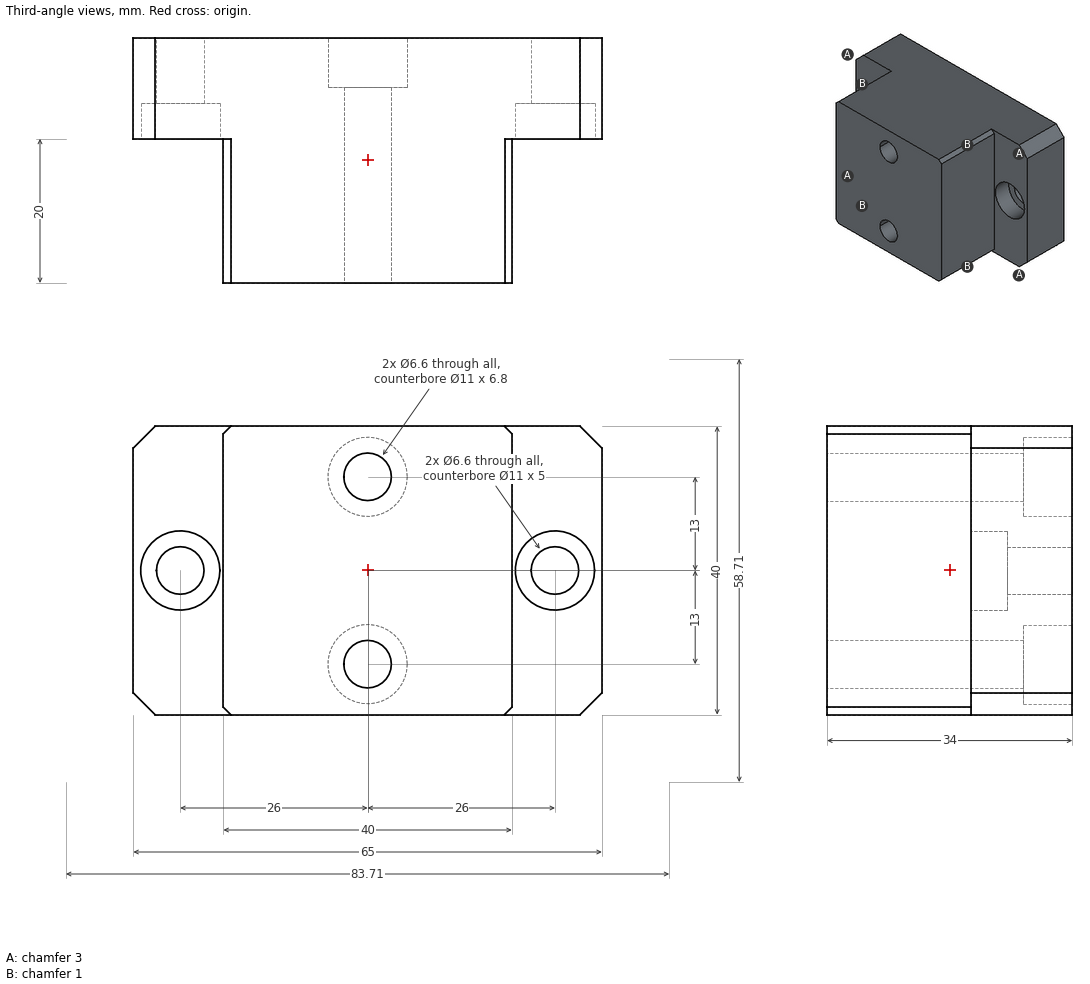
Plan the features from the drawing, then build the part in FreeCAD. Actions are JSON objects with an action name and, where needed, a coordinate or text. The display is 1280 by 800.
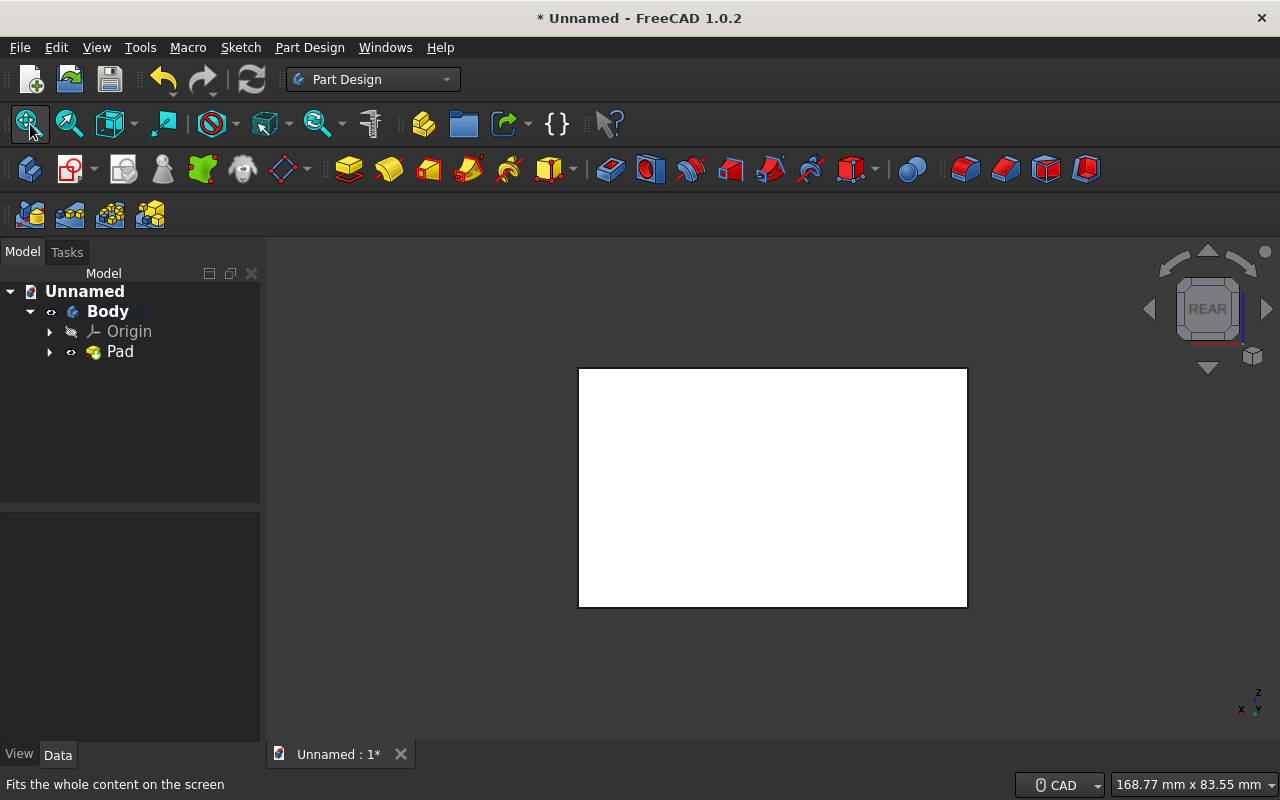
{"action": "left_click", "coordinate": [717, 487]}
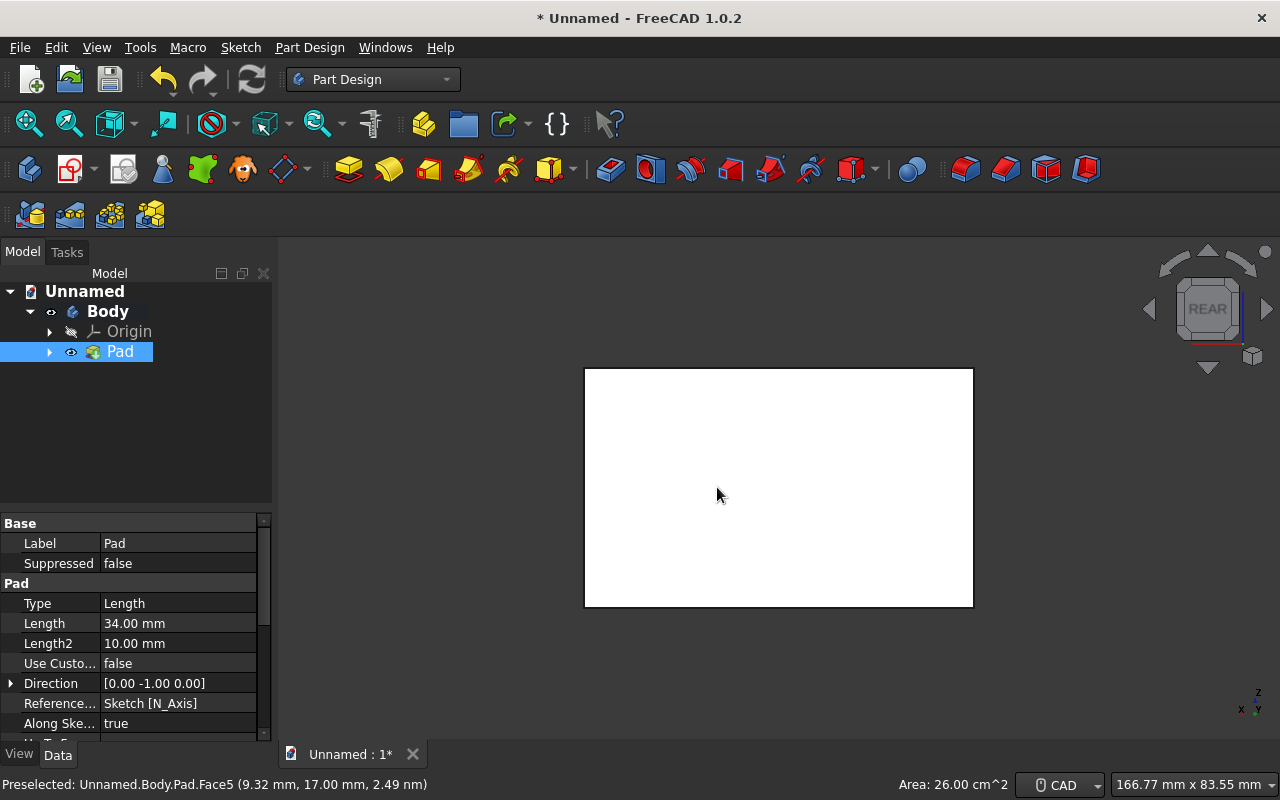
{"action": "left_click", "coordinate": [70, 170]}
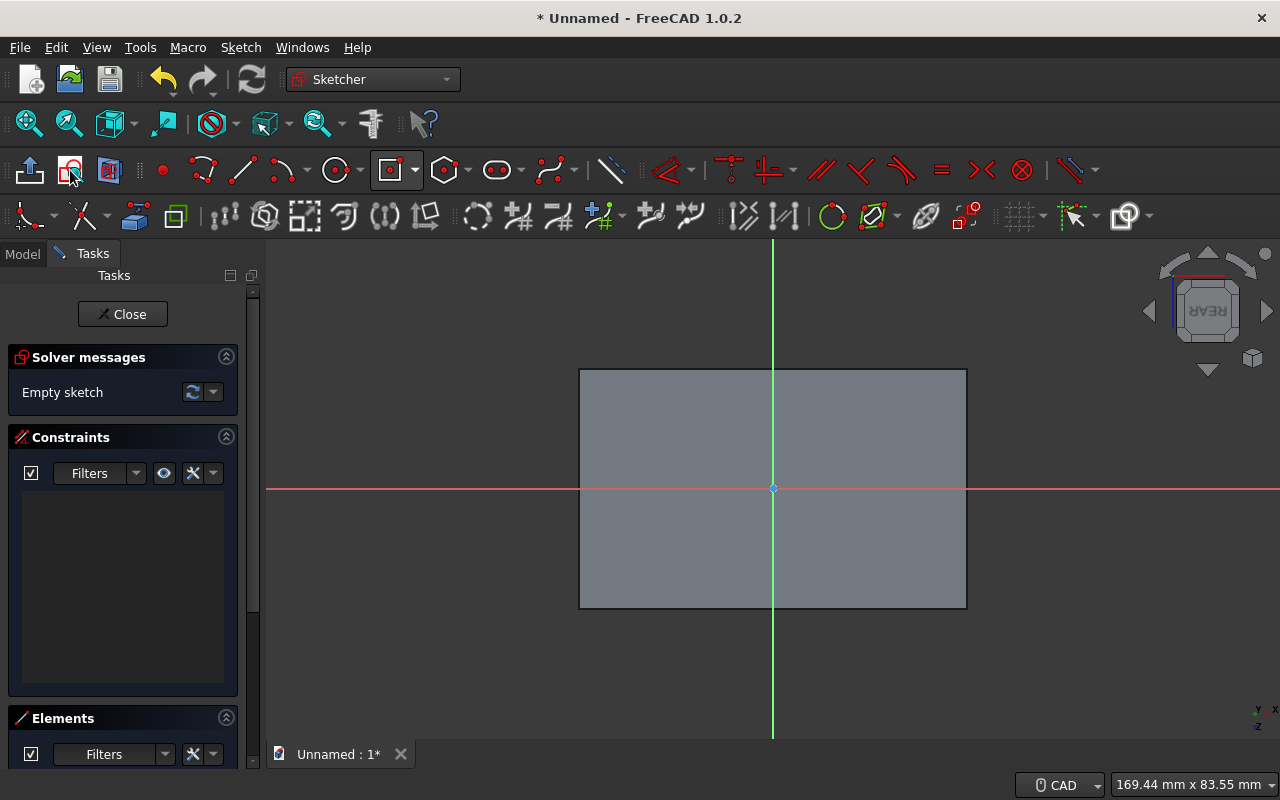
{"action": "scroll", "coordinate": [912, 489], "scroll_direction": "up", "scroll_amount": 2}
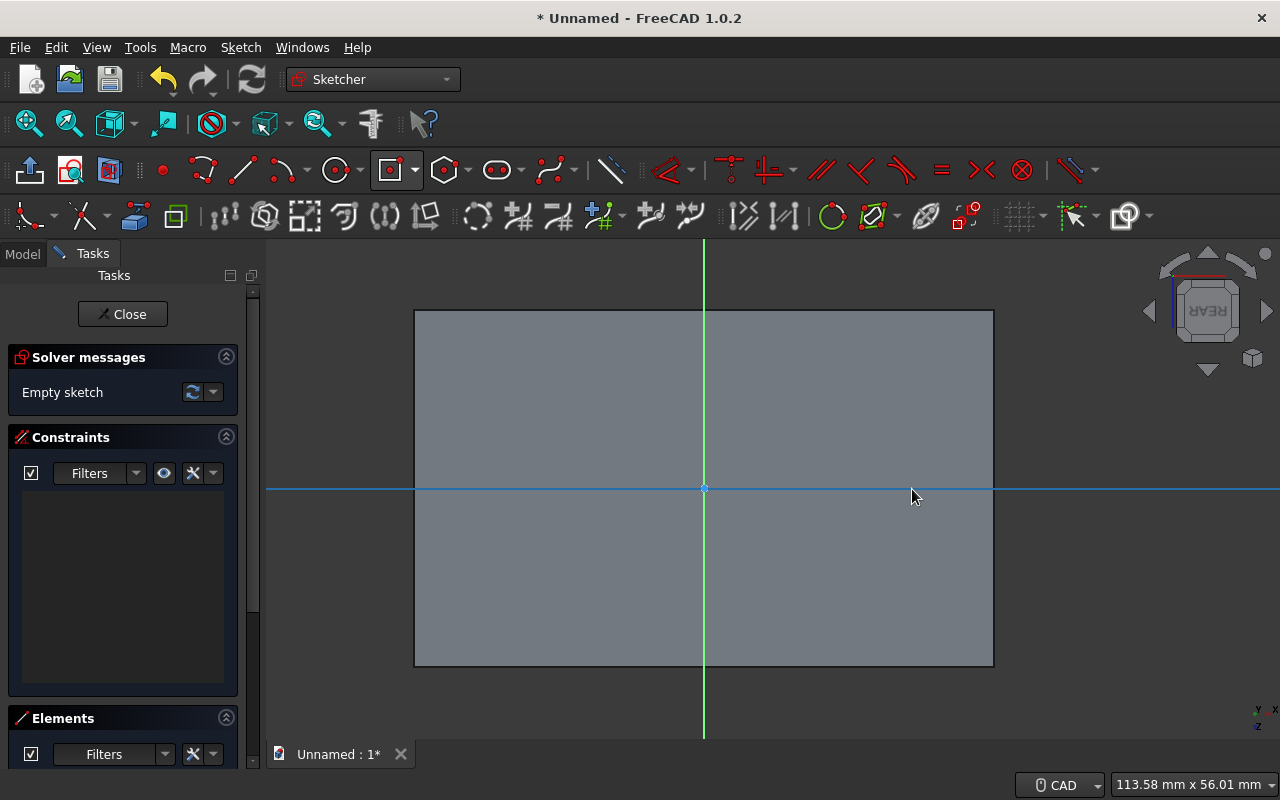
{"action": "left_click", "coordinate": [336, 170]}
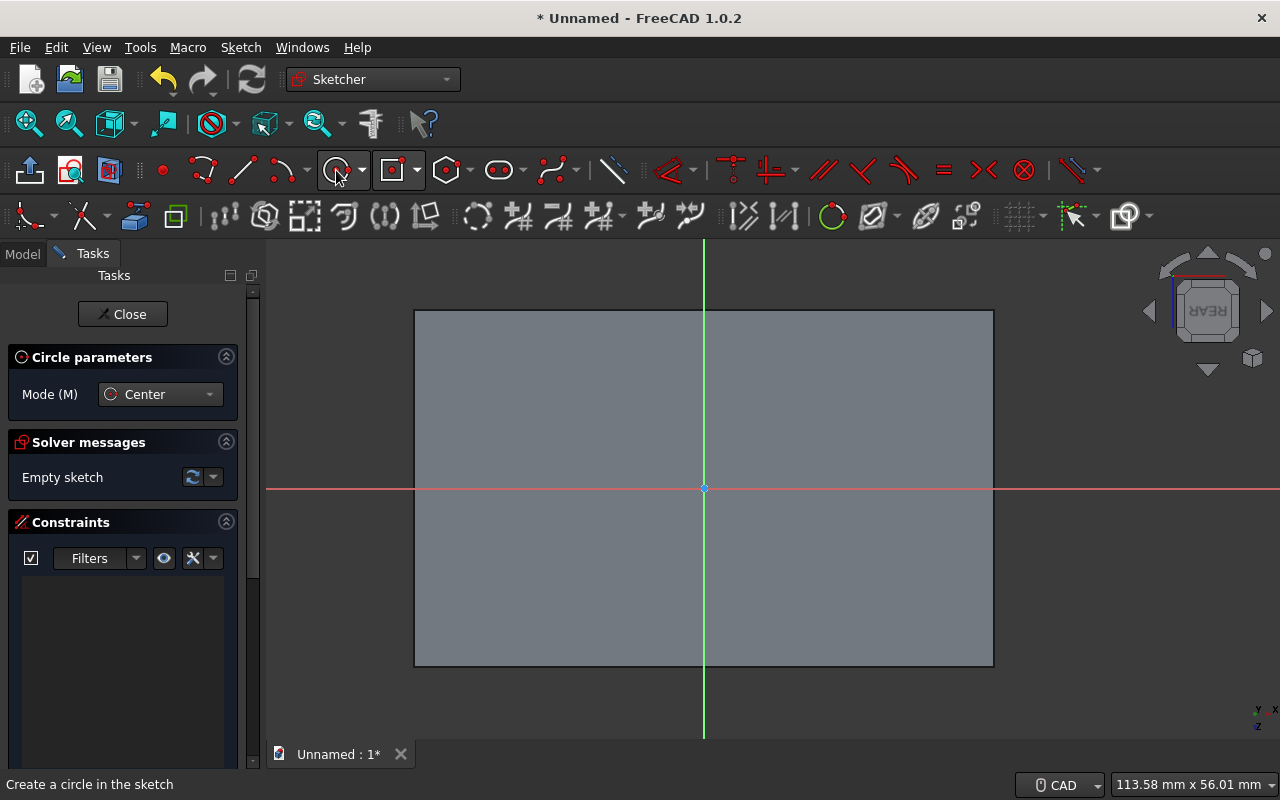
{"action": "left_click", "coordinate": [704, 605]}
{"action": "left_click", "coordinate": [725, 584]}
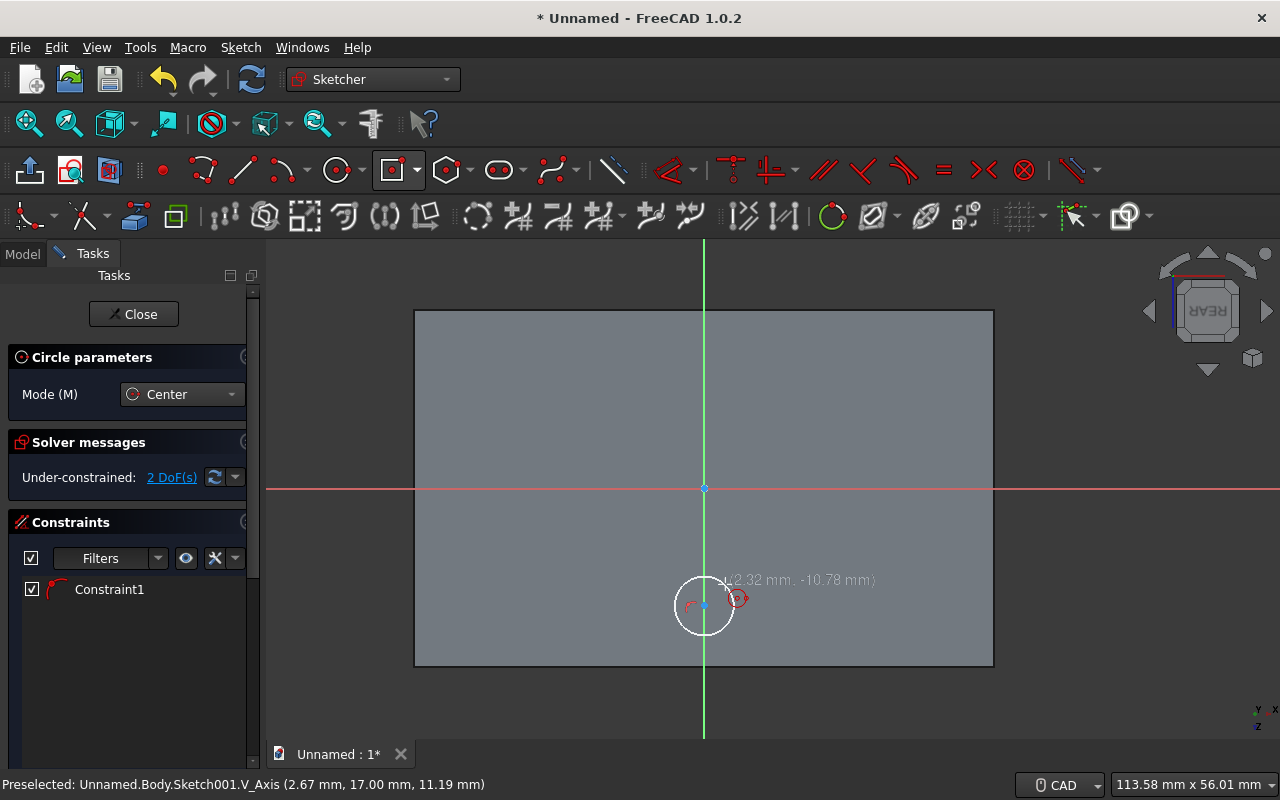
{"action": "left_click", "coordinate": [704, 373]}
{"action": "left_click", "coordinate": [725, 352]}
{"action": "key", "text": "Escape"}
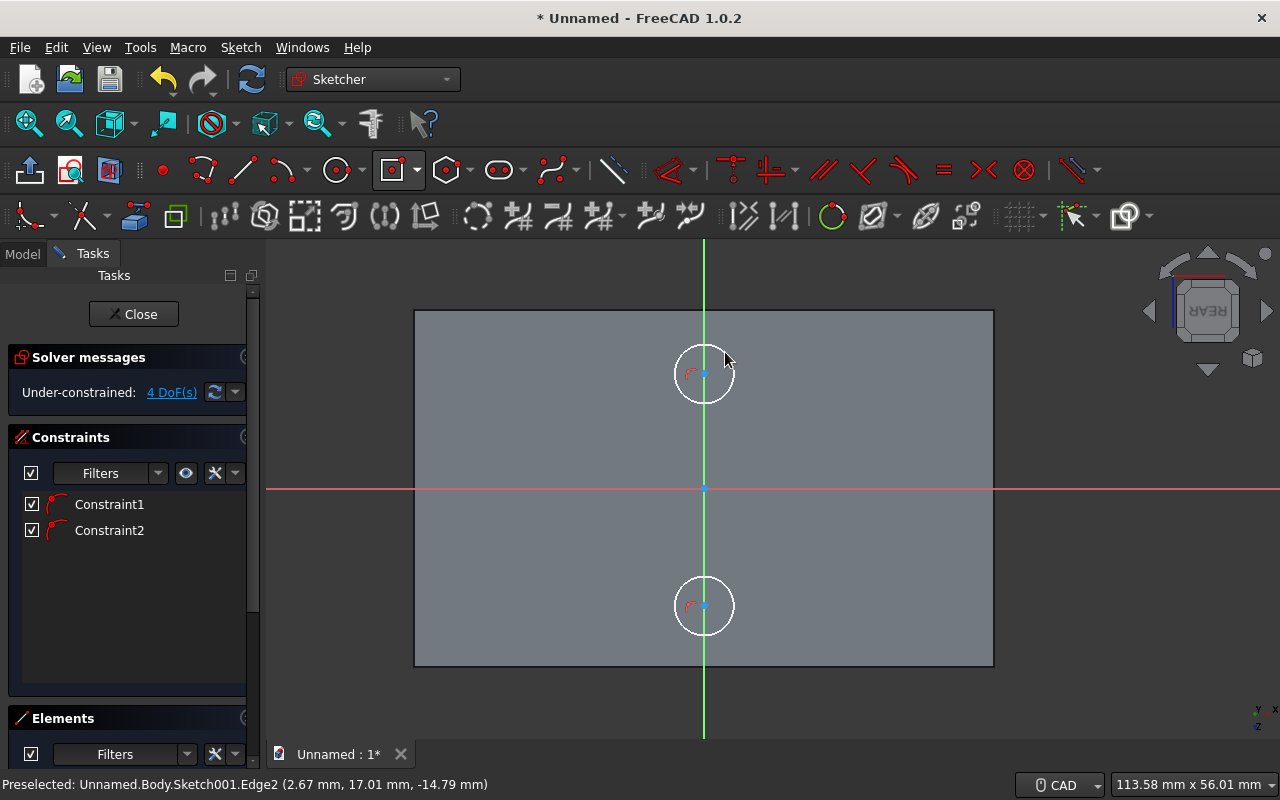
{"action": "left_click", "coordinate": [725, 585]}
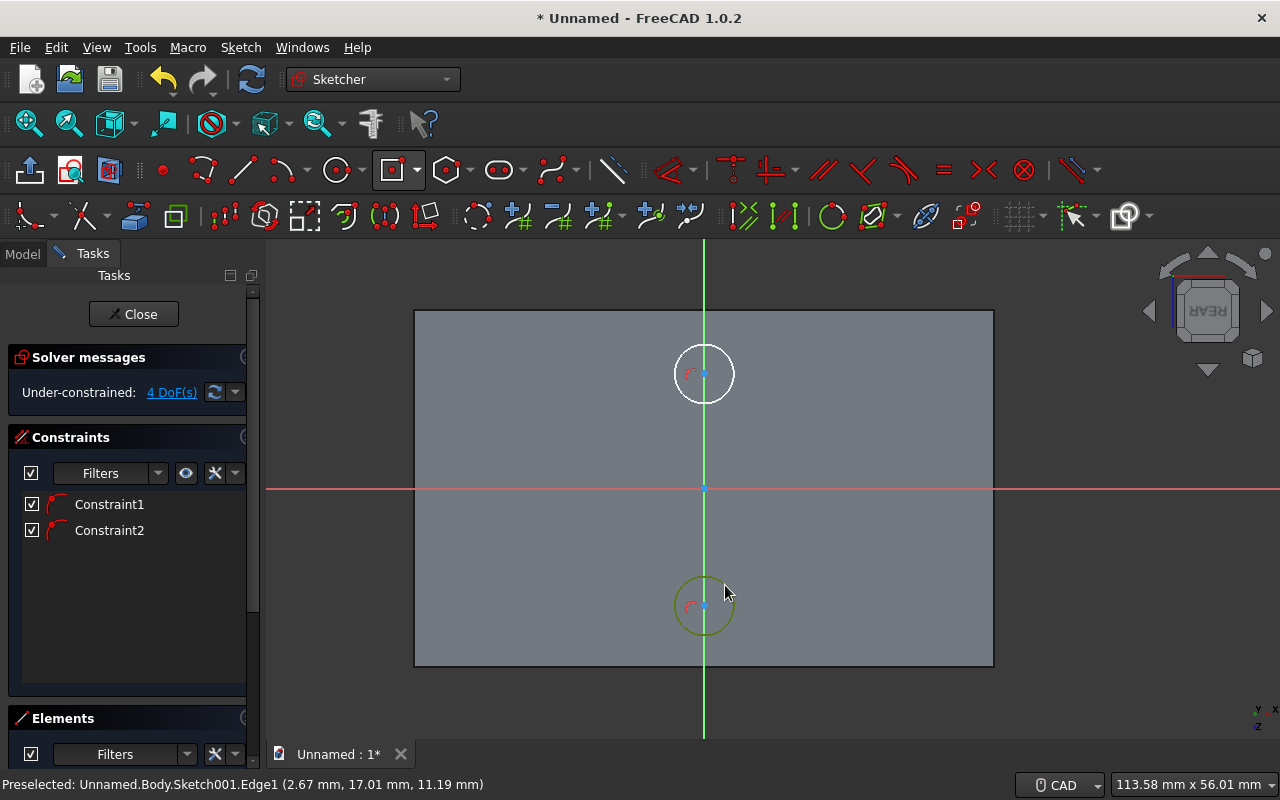
{"action": "left_click", "coordinate": [725, 353]}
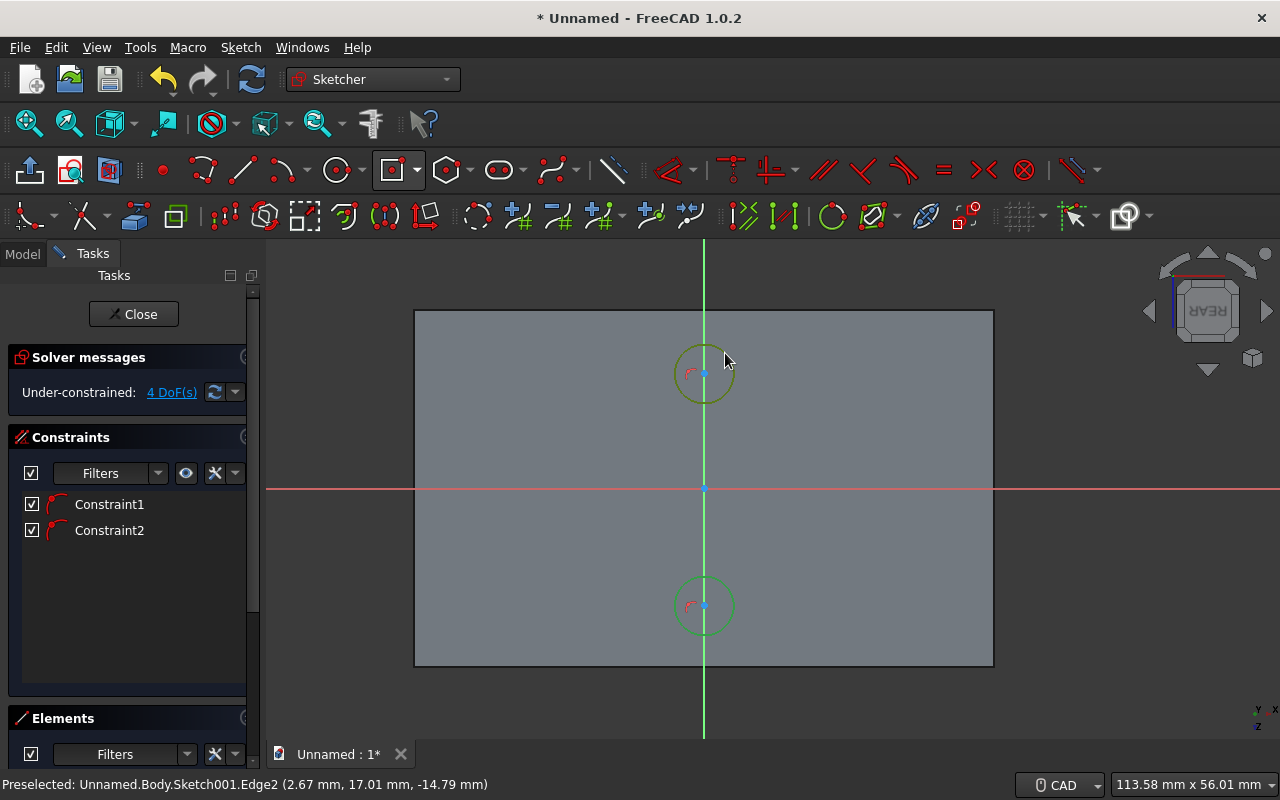
{"action": "left_click", "coordinate": [944, 170]}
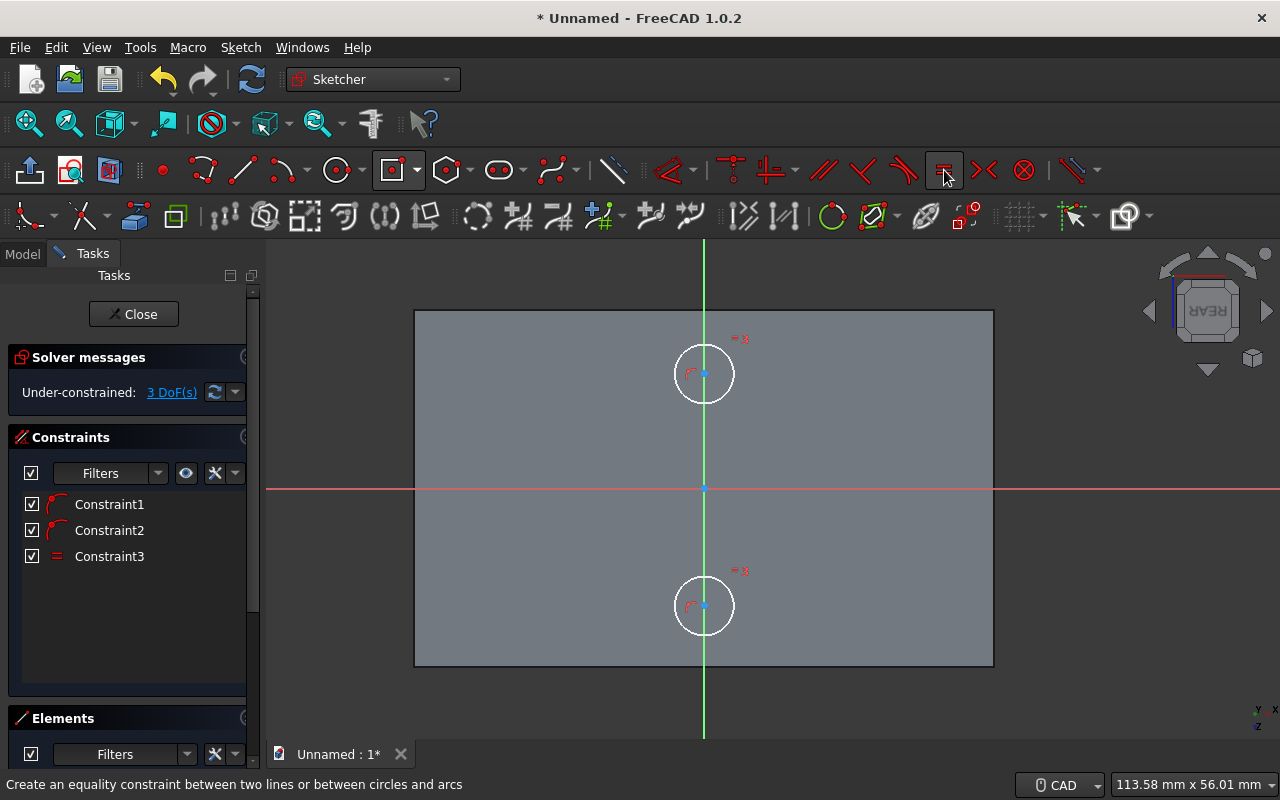
{"action": "left_click", "coordinate": [668, 170]}